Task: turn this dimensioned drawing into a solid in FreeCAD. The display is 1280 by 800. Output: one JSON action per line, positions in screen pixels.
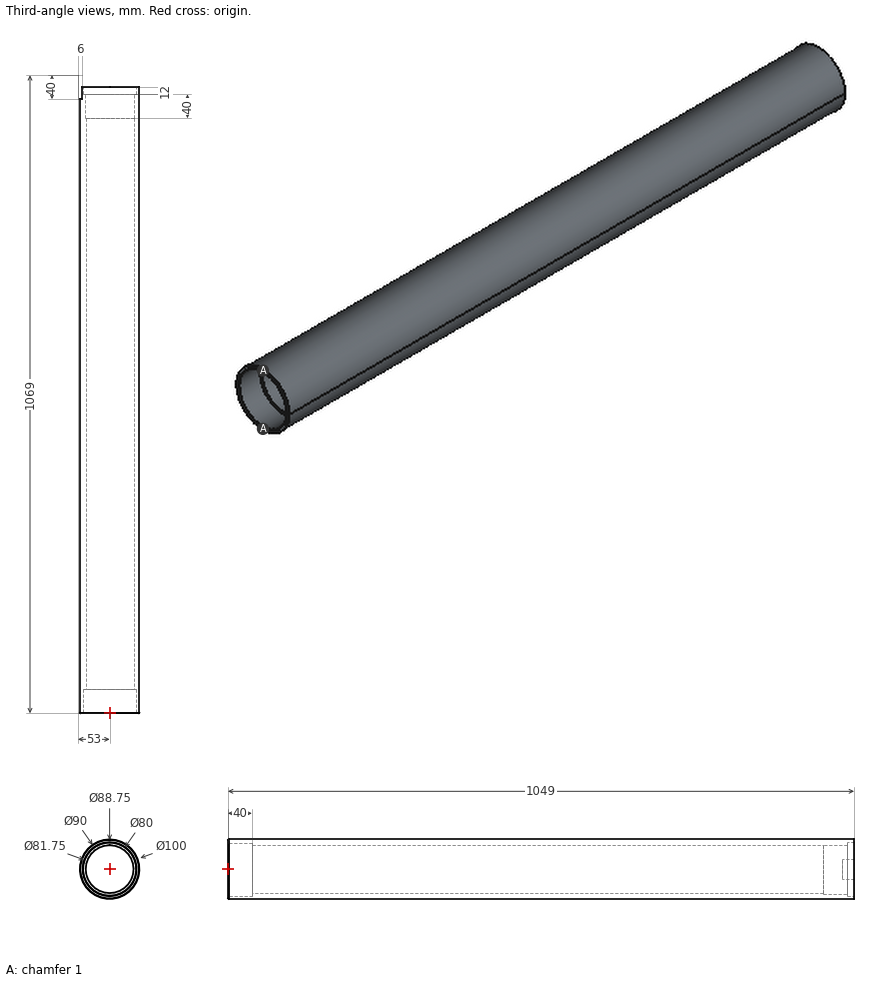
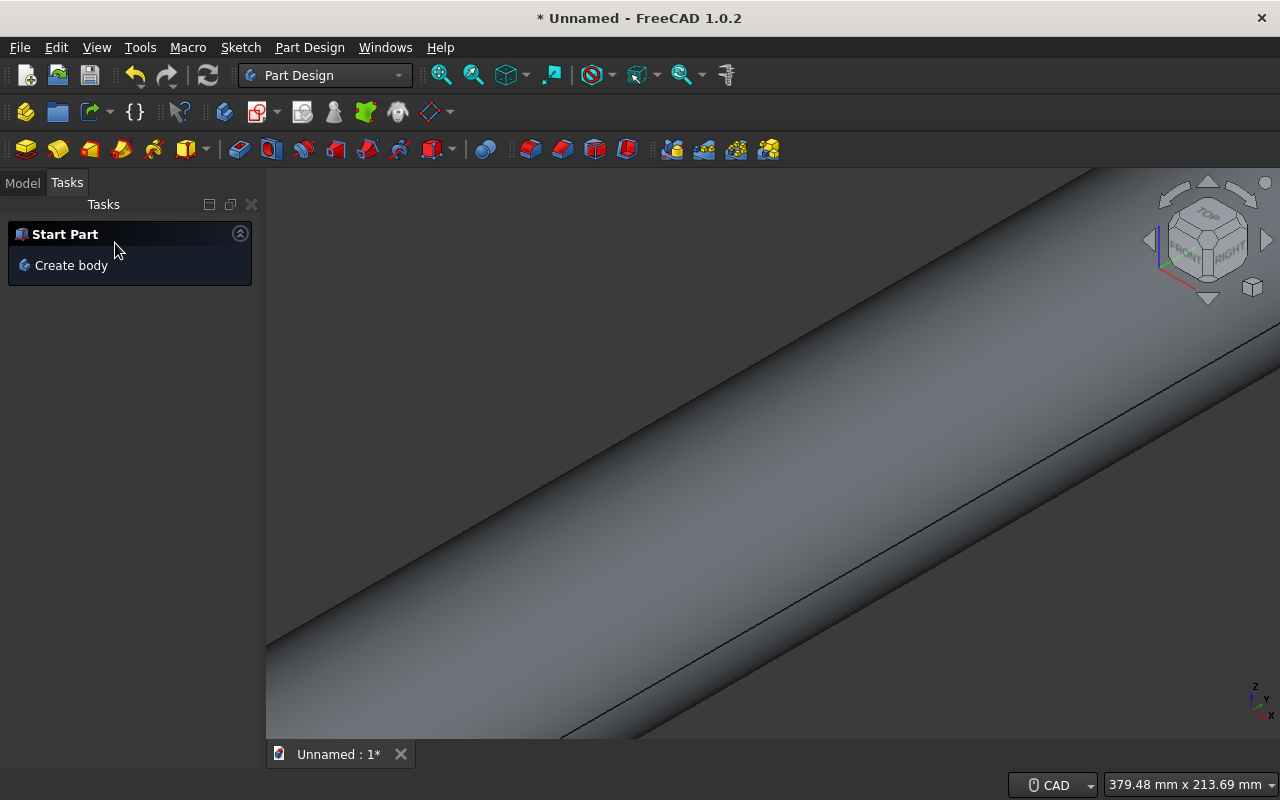
{"action": "left_click", "coordinate": [442, 76]}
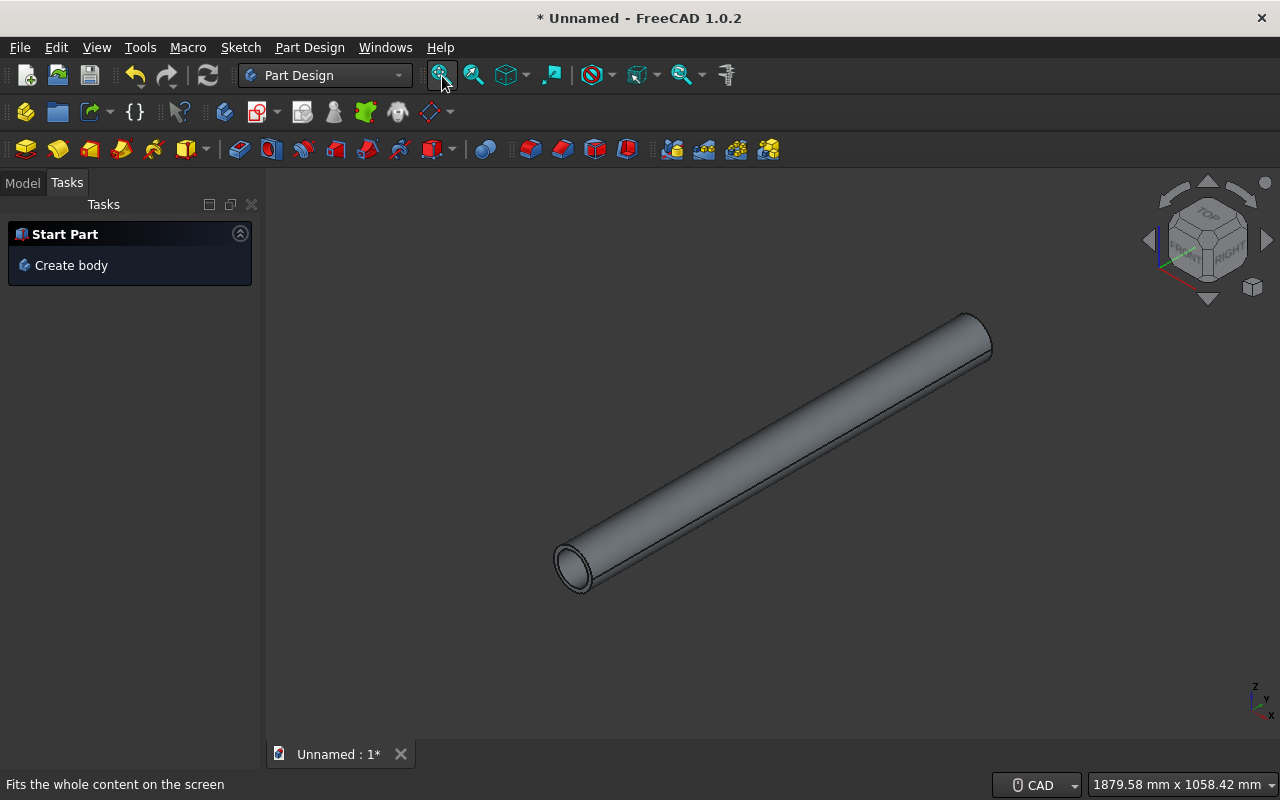
{"action": "scroll", "coordinate": [557, 565], "scroll_direction": "up", "scroll_amount": 8}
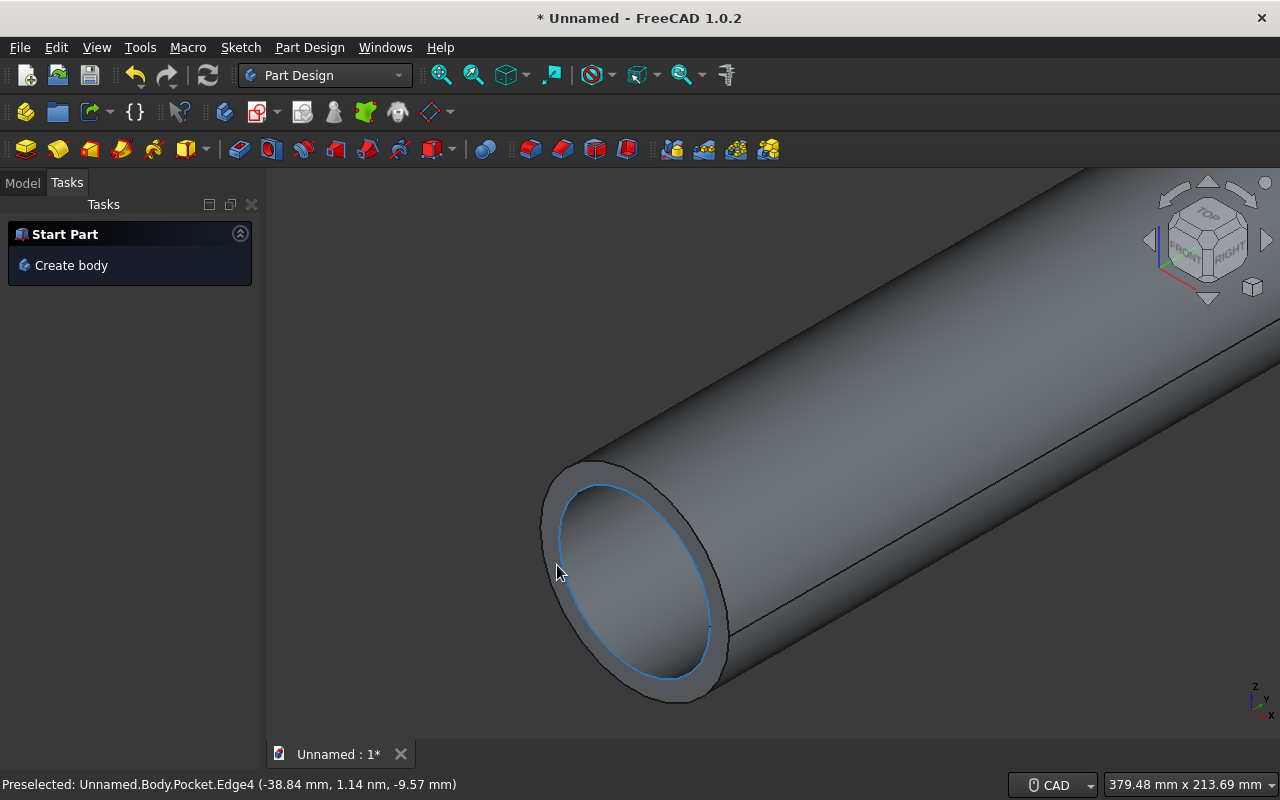
{"action": "left_click", "coordinate": [554, 566]}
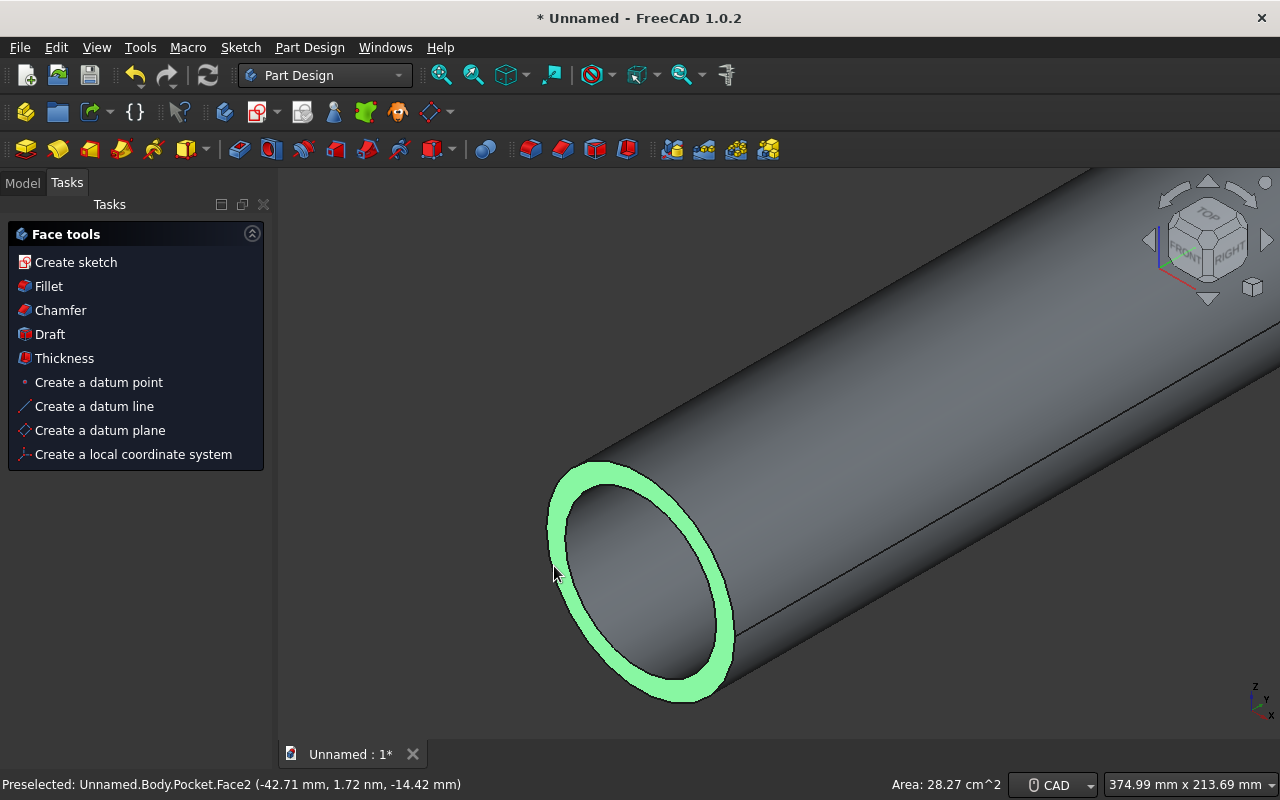
{"action": "left_click", "coordinate": [258, 112]}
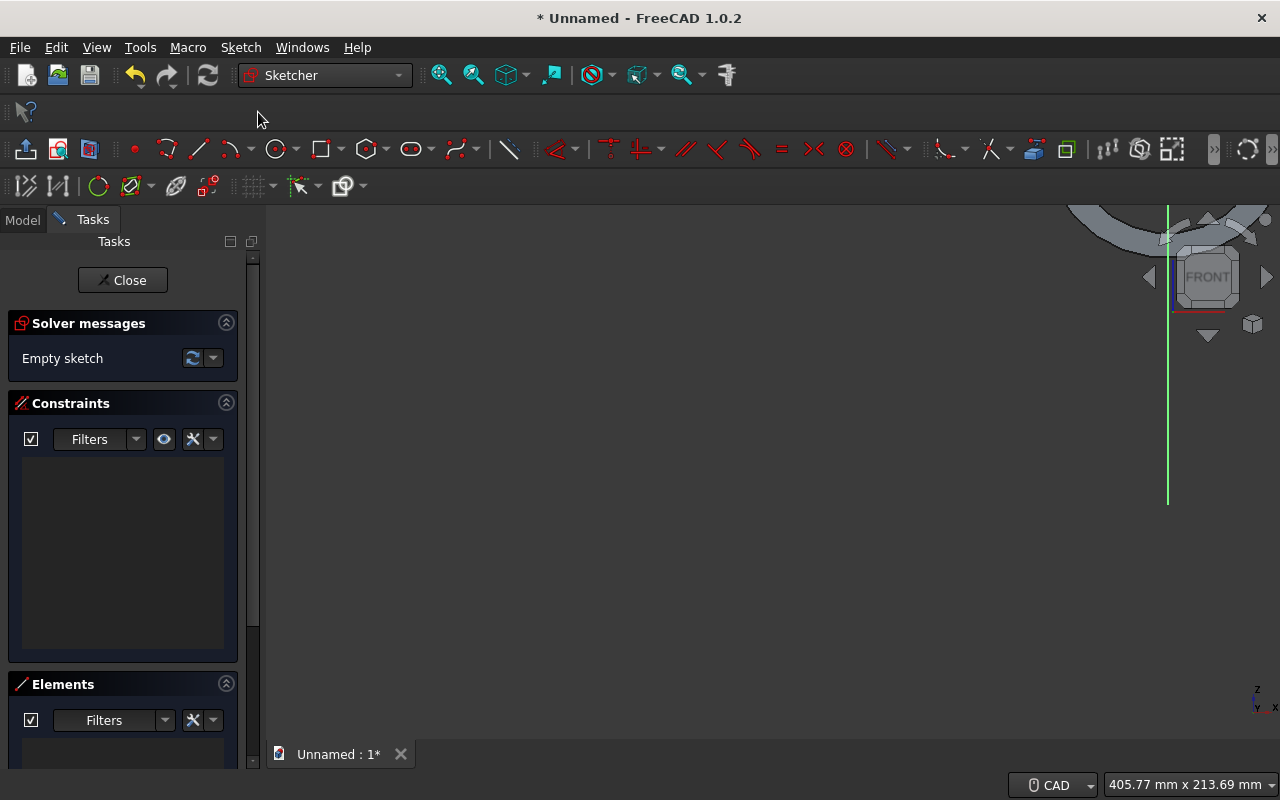
{"action": "scroll", "coordinate": [704, 472], "scroll_direction": "down", "scroll_amount": 5}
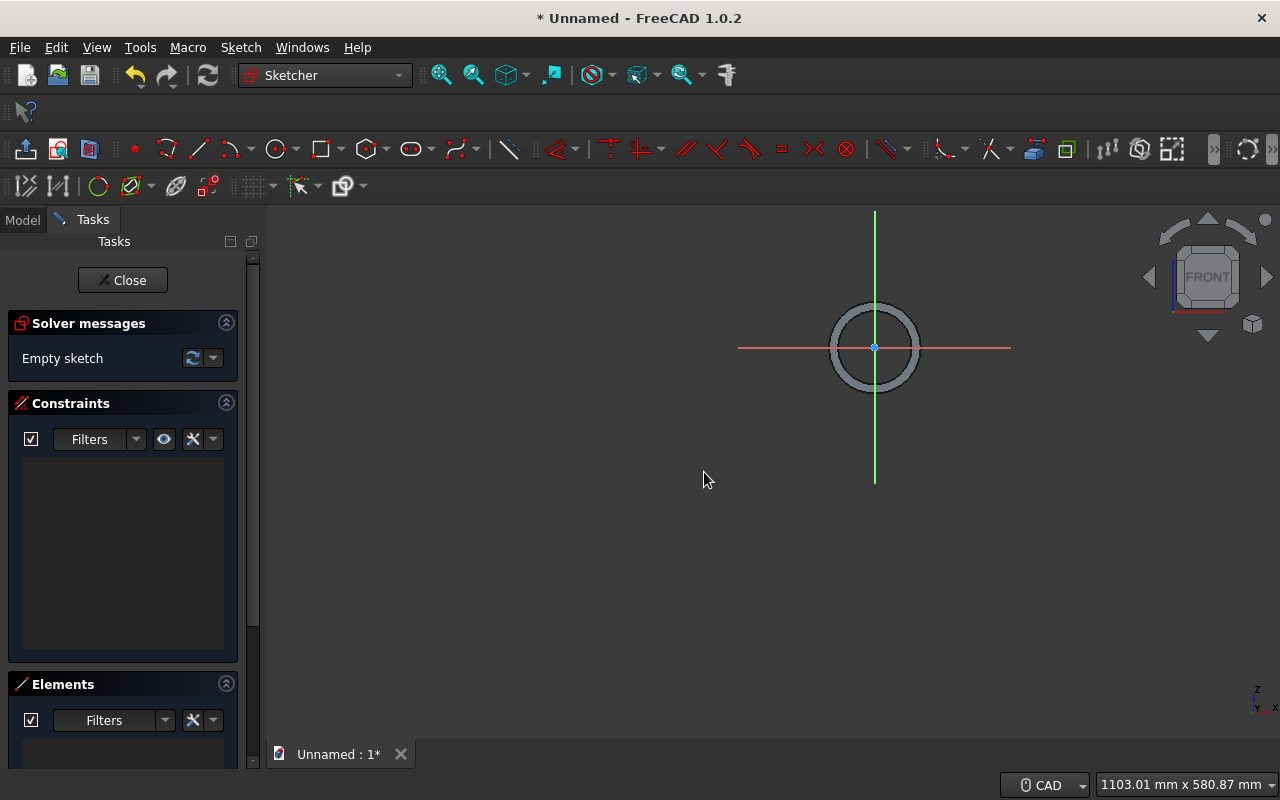
{"action": "scroll", "coordinate": [931, 307], "scroll_direction": "up", "scroll_amount": 7}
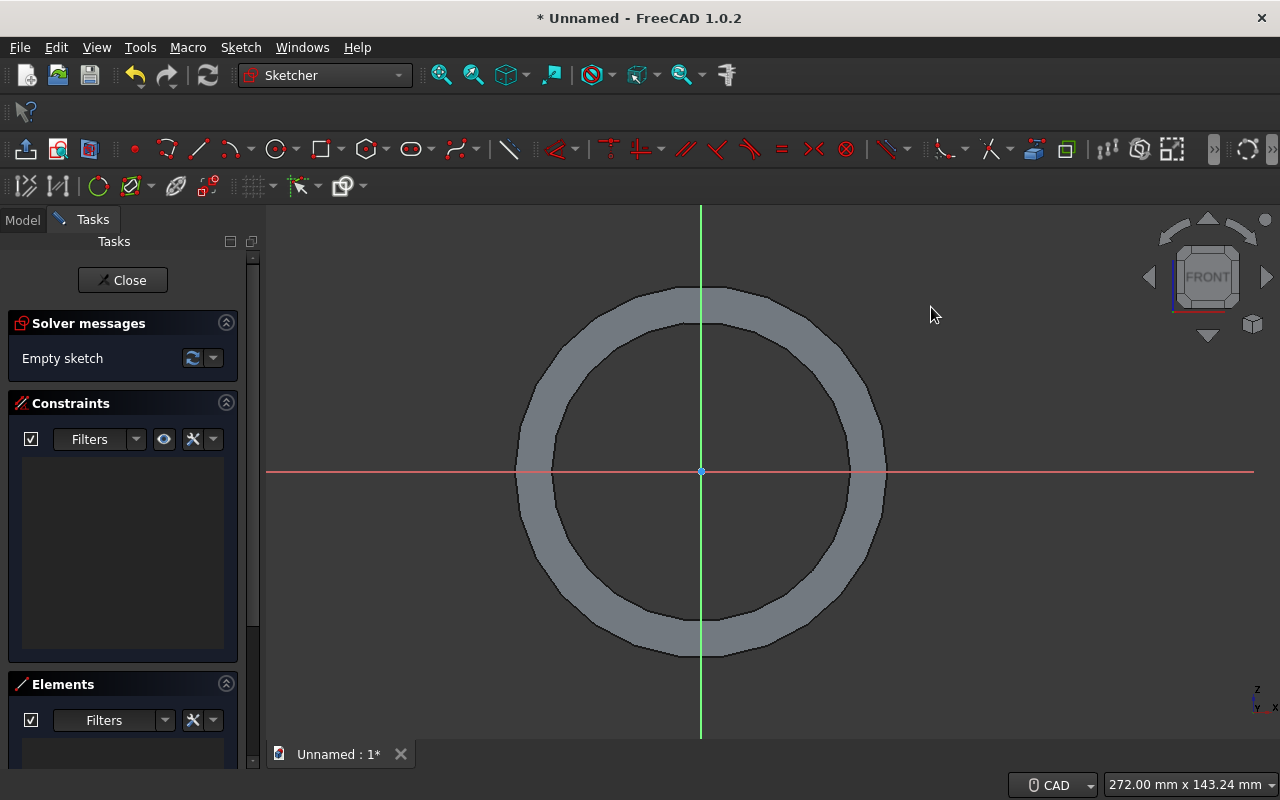
{"action": "left_click", "coordinate": [276, 150]}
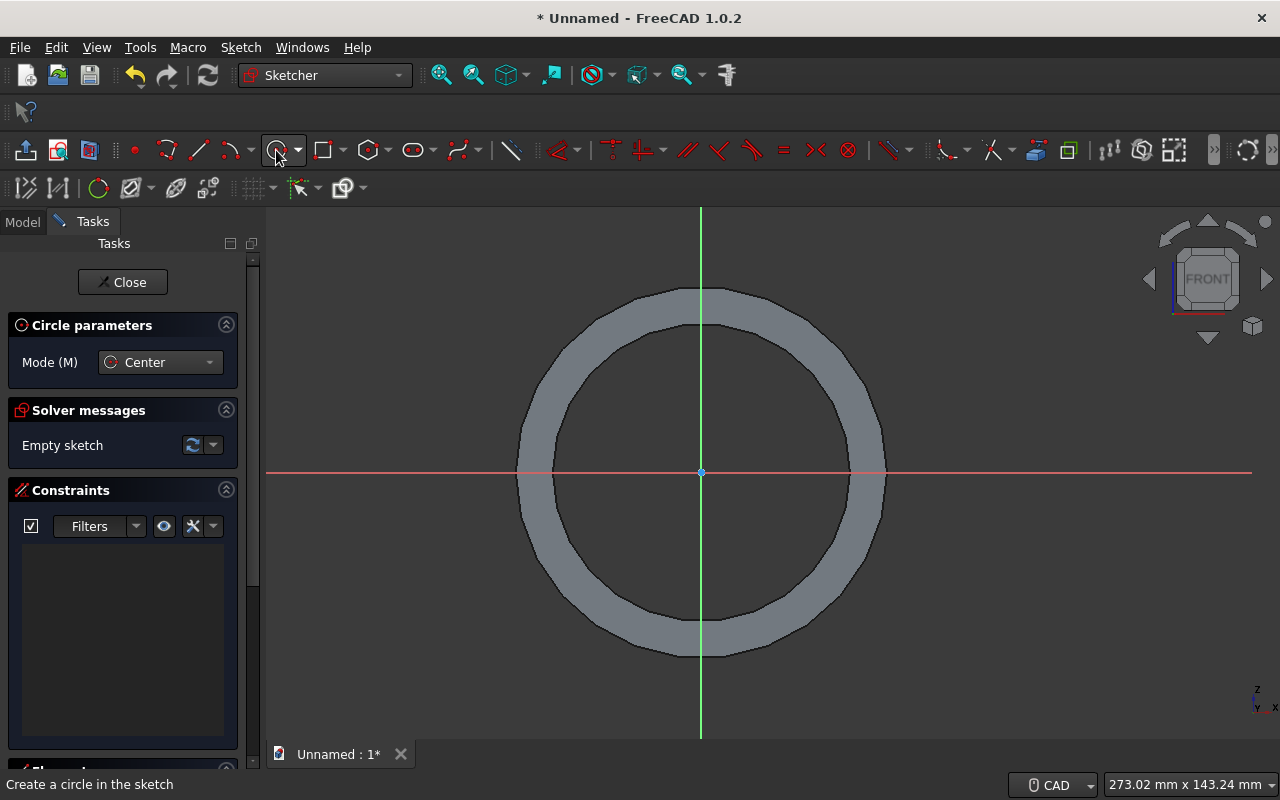
{"action": "left_click", "coordinate": [701, 473]}
{"action": "mouse_move", "coordinate": [818, 356]}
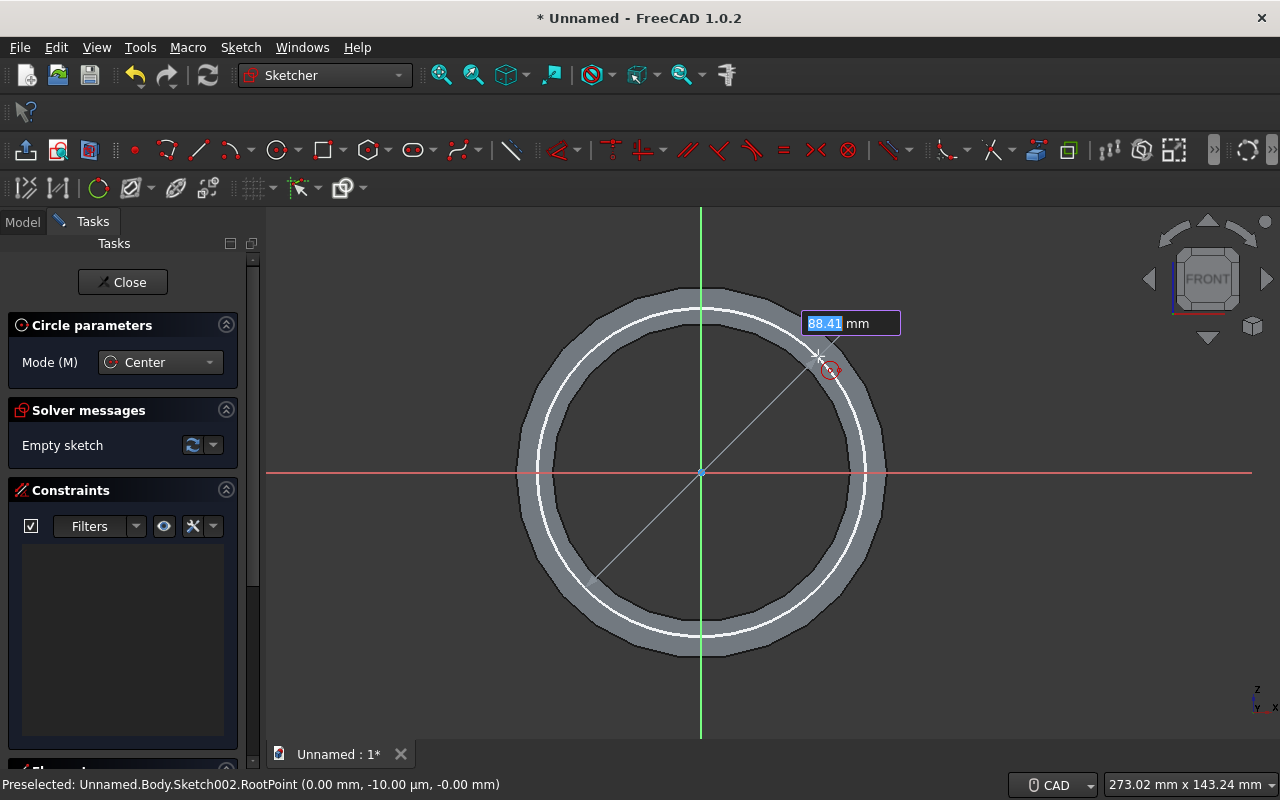
{"action": "type", "text": "88.75"}
{"action": "key", "text": "Return"}
{"action": "key", "text": "Escape"}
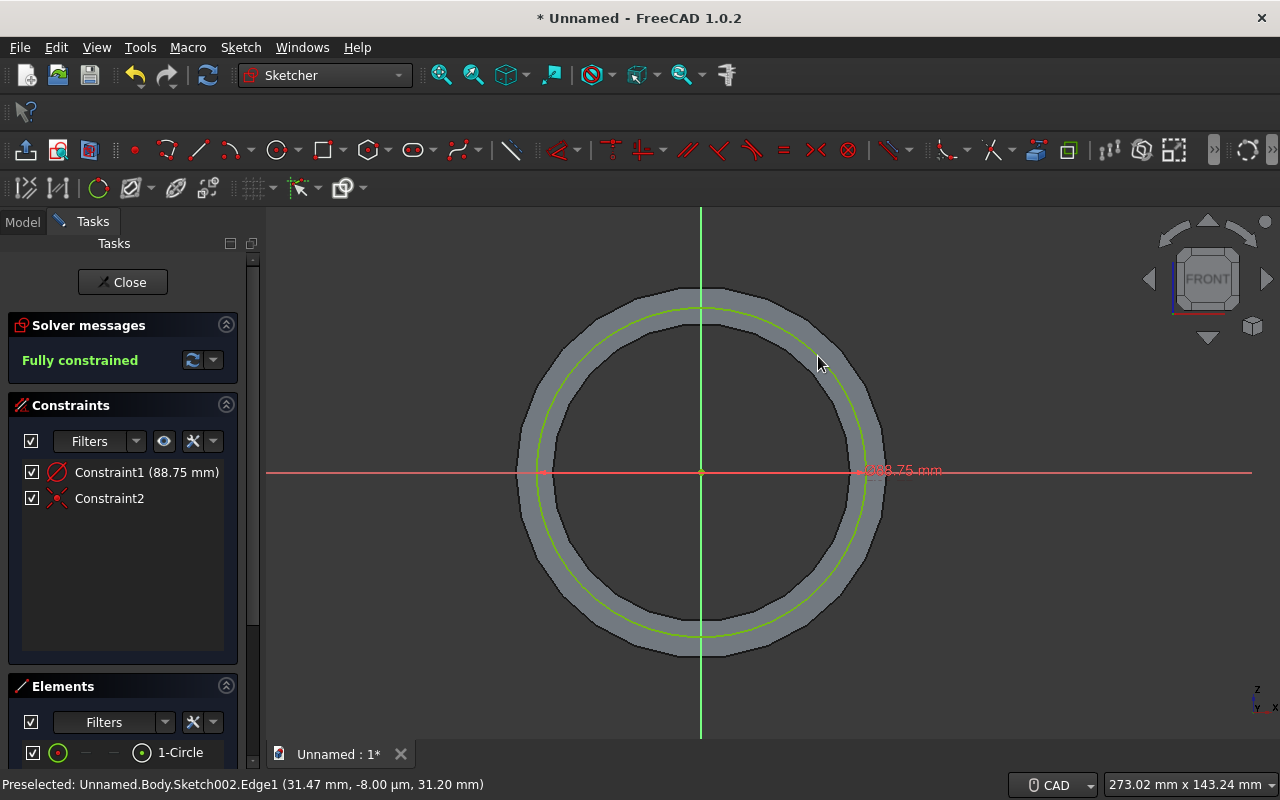
{"action": "left_click", "coordinate": [123, 282]}